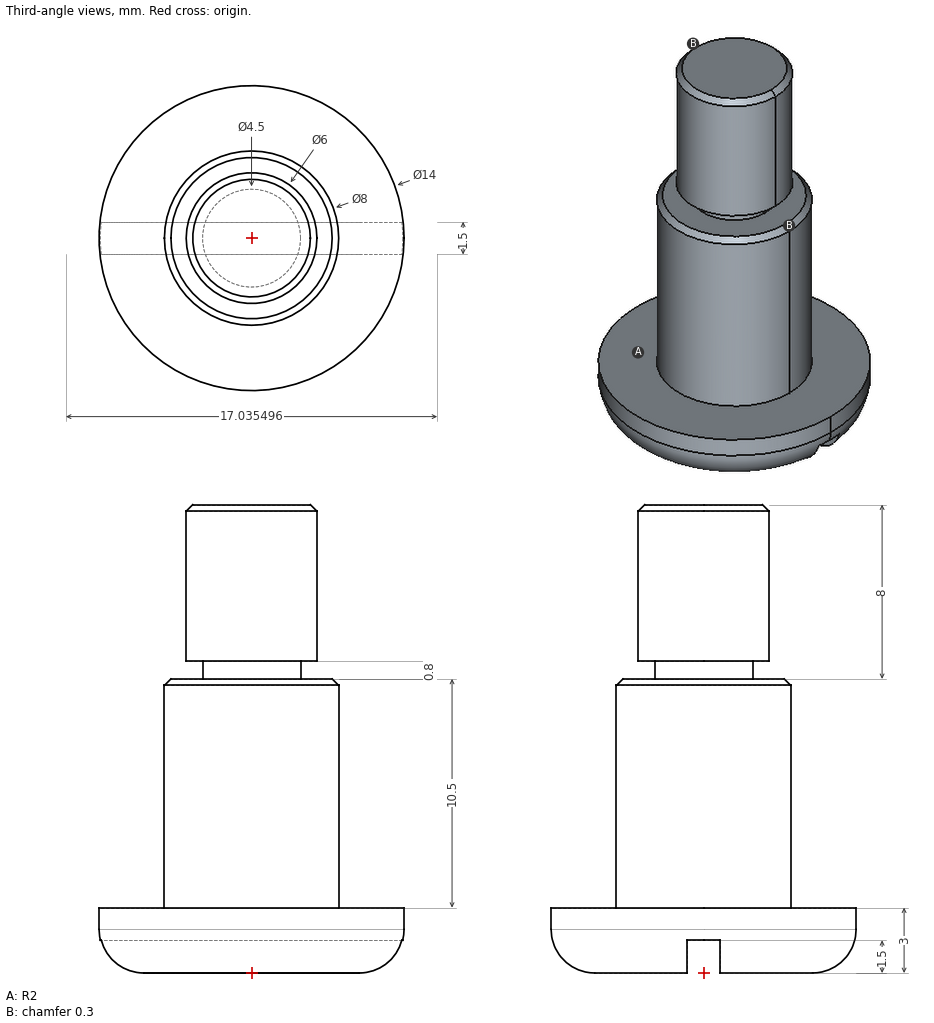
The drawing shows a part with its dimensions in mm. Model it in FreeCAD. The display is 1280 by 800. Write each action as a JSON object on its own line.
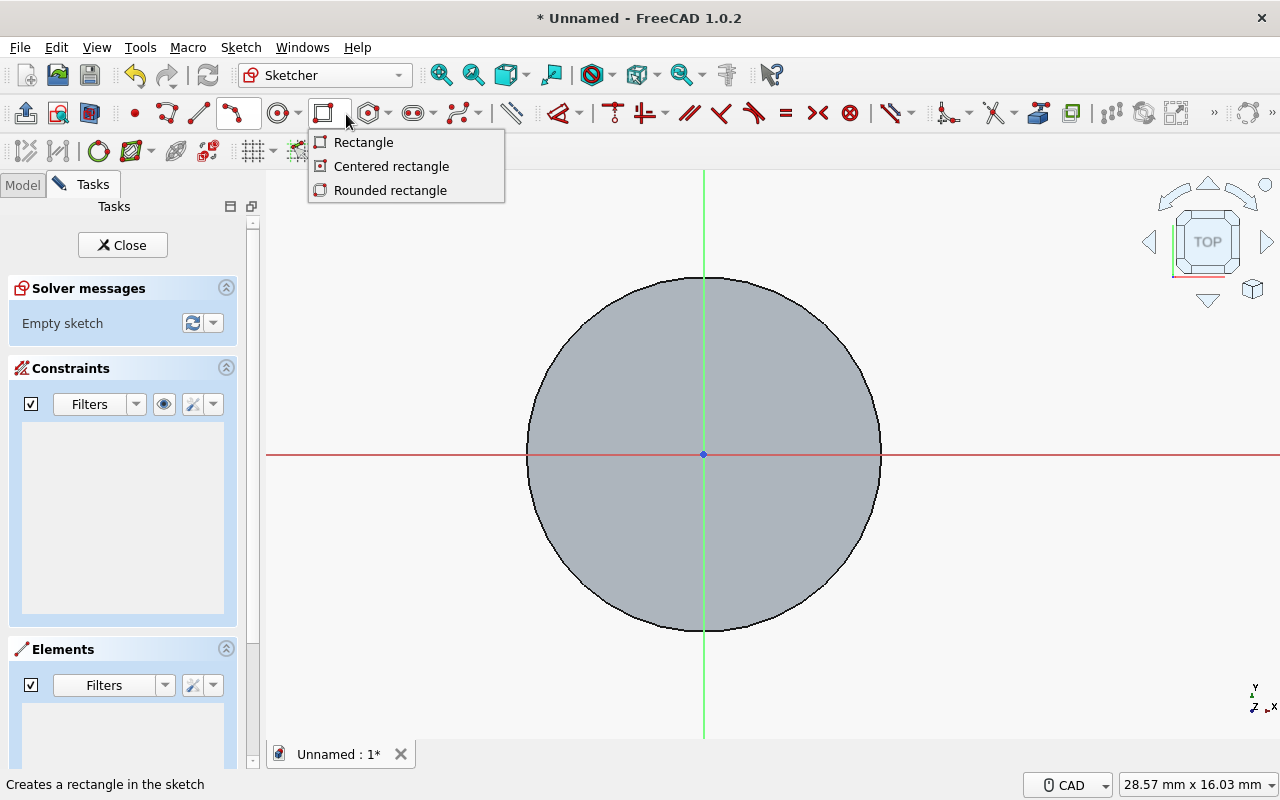
{"action": "left_click", "coordinate": [406, 166]}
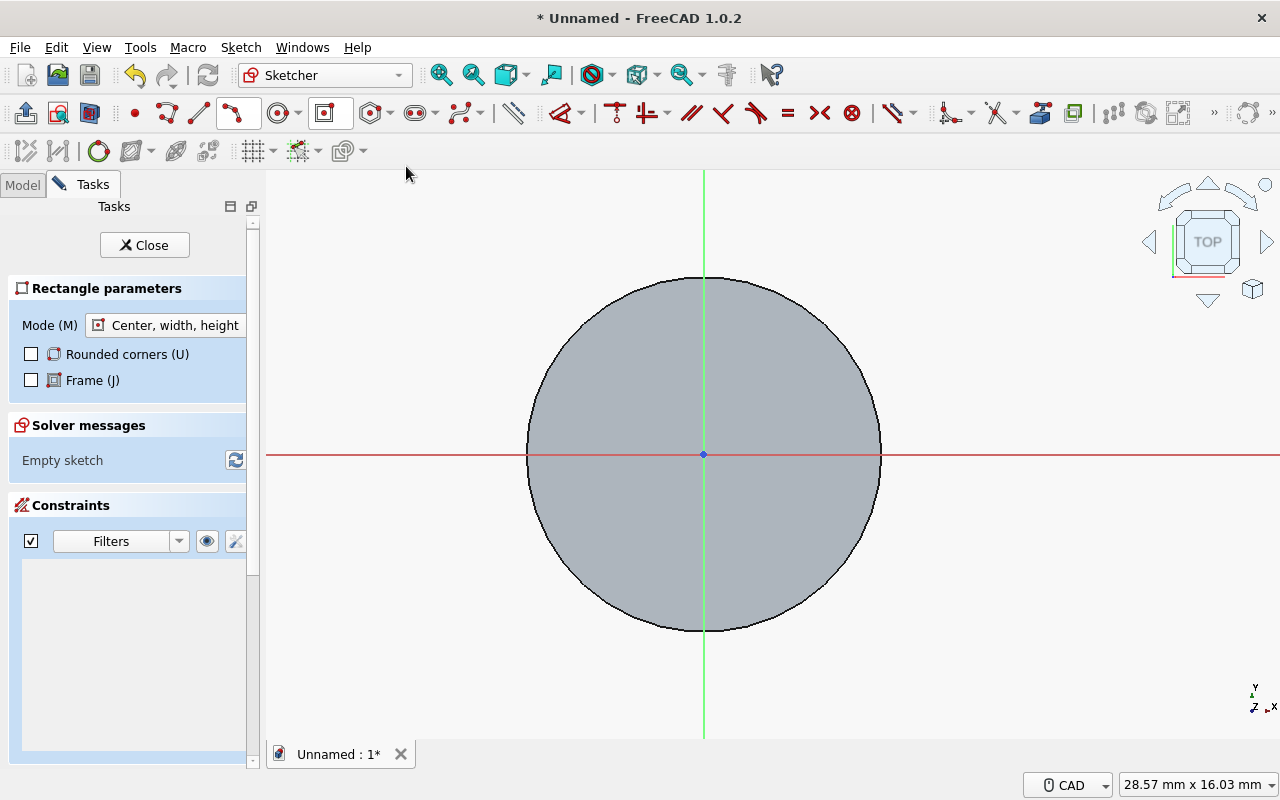
{"action": "left_click", "coordinate": [704, 454]}
{"action": "left_click", "coordinate": [1006, 428]}
{"action": "key", "text": "Escape"}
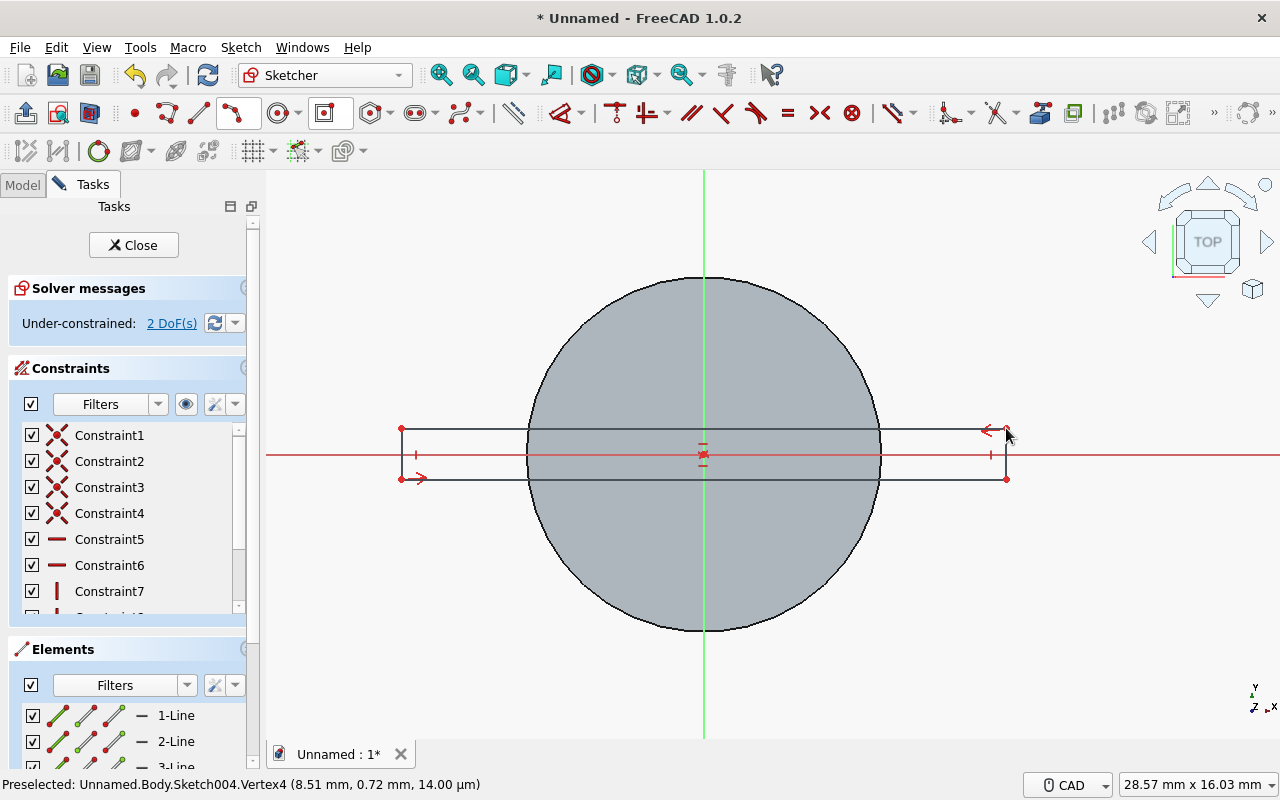
{"action": "left_click", "coordinate": [560, 114]}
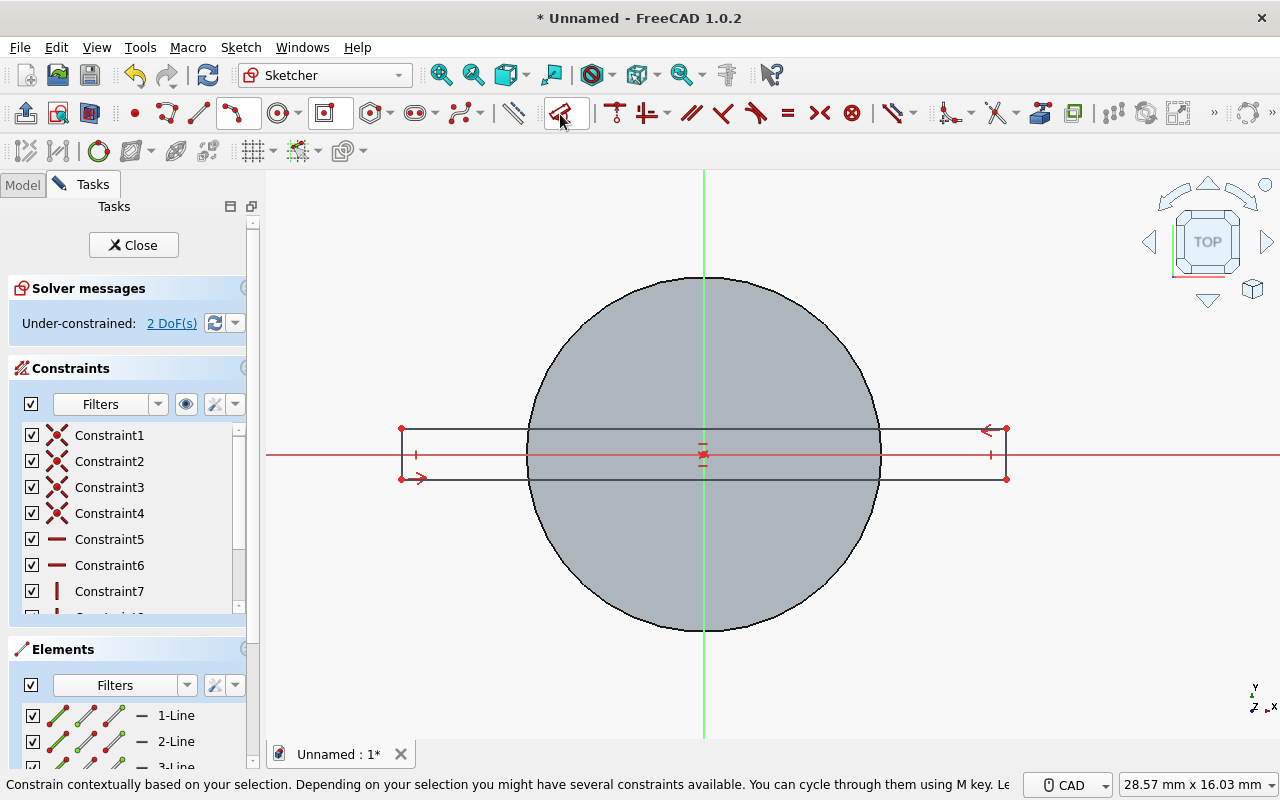
{"action": "scroll", "coordinate": [1006, 465], "scroll_direction": "up", "scroll_amount": 2}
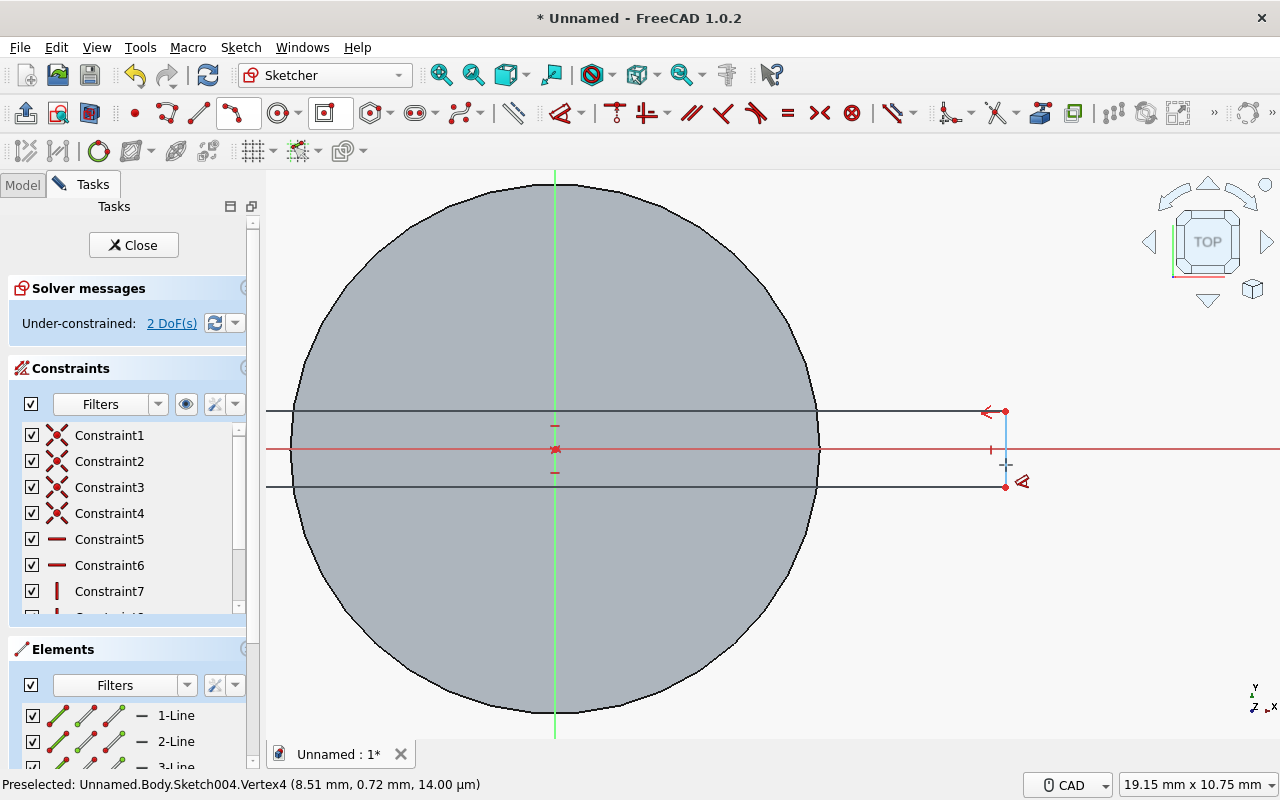
{"action": "left_click", "coordinate": [1006, 464]}
{"action": "left_click", "coordinate": [1040, 432]}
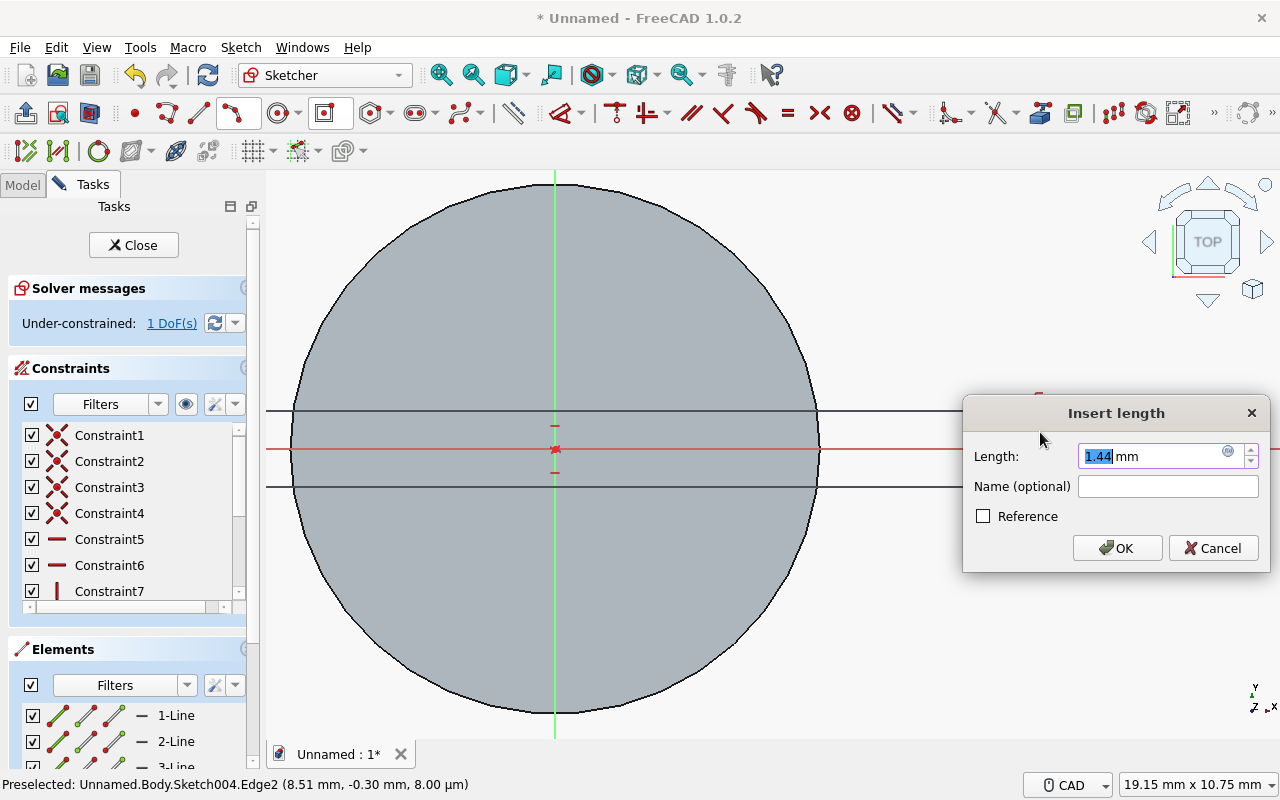
{"action": "type", "text": "1.5"}
{"action": "key", "text": "Return"}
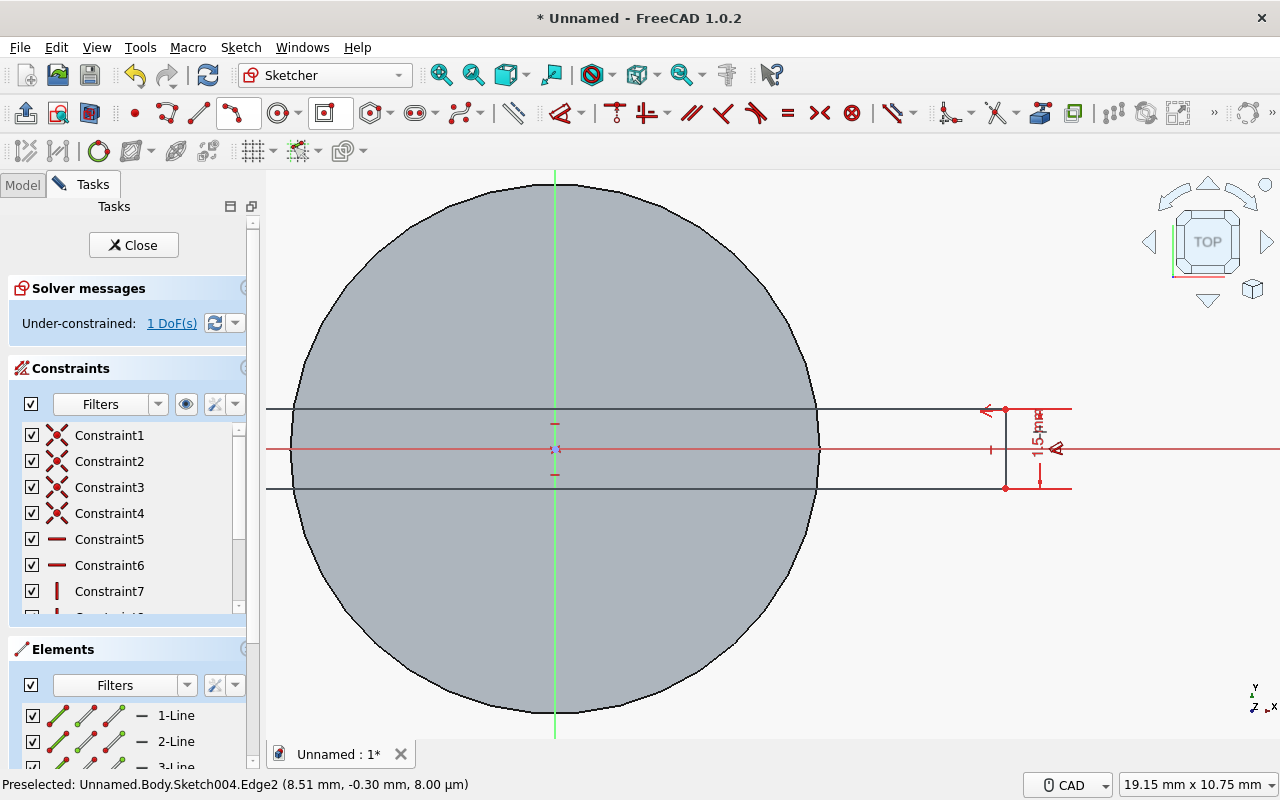
{"action": "left_click", "coordinate": [375, 489]}
{"action": "left_click", "coordinate": [650, 523]}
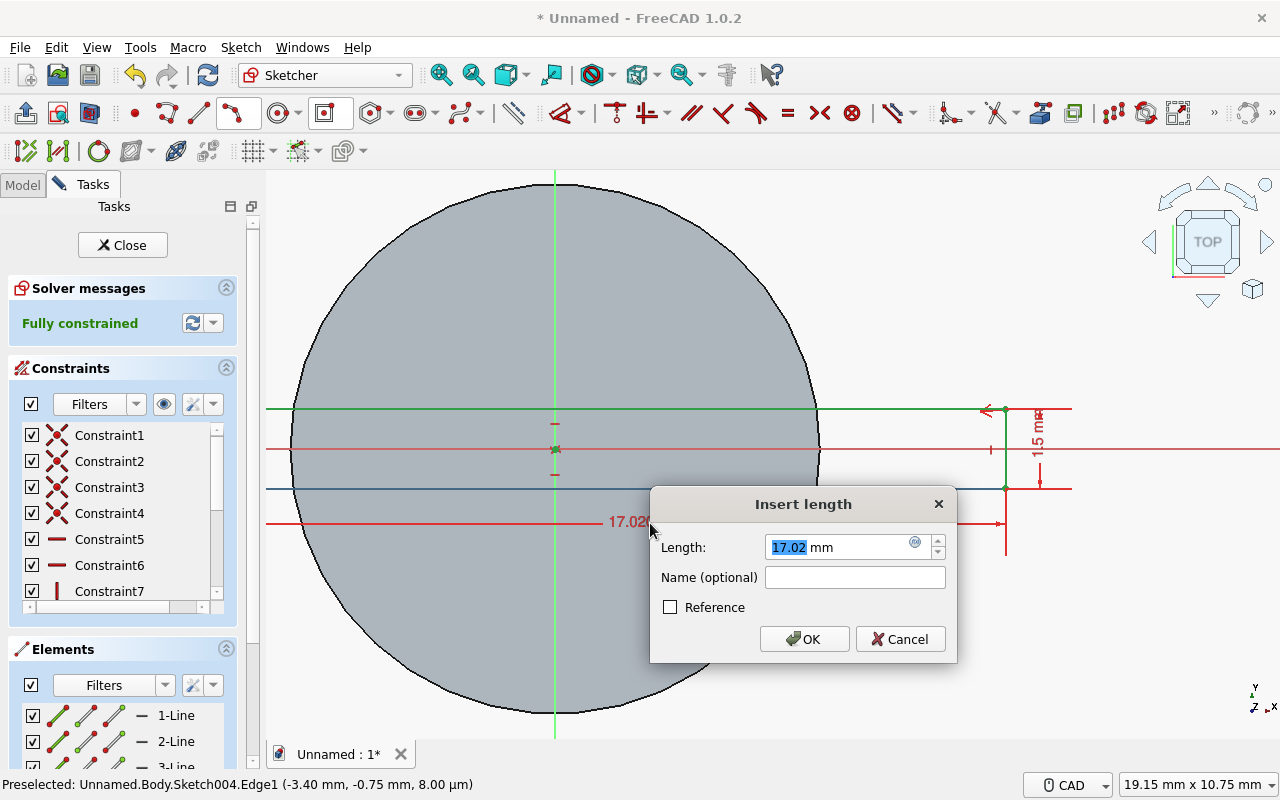
{"action": "type", "text": "17.035496"}
{"action": "key", "text": "Return"}
{"action": "key", "text": "Escape"}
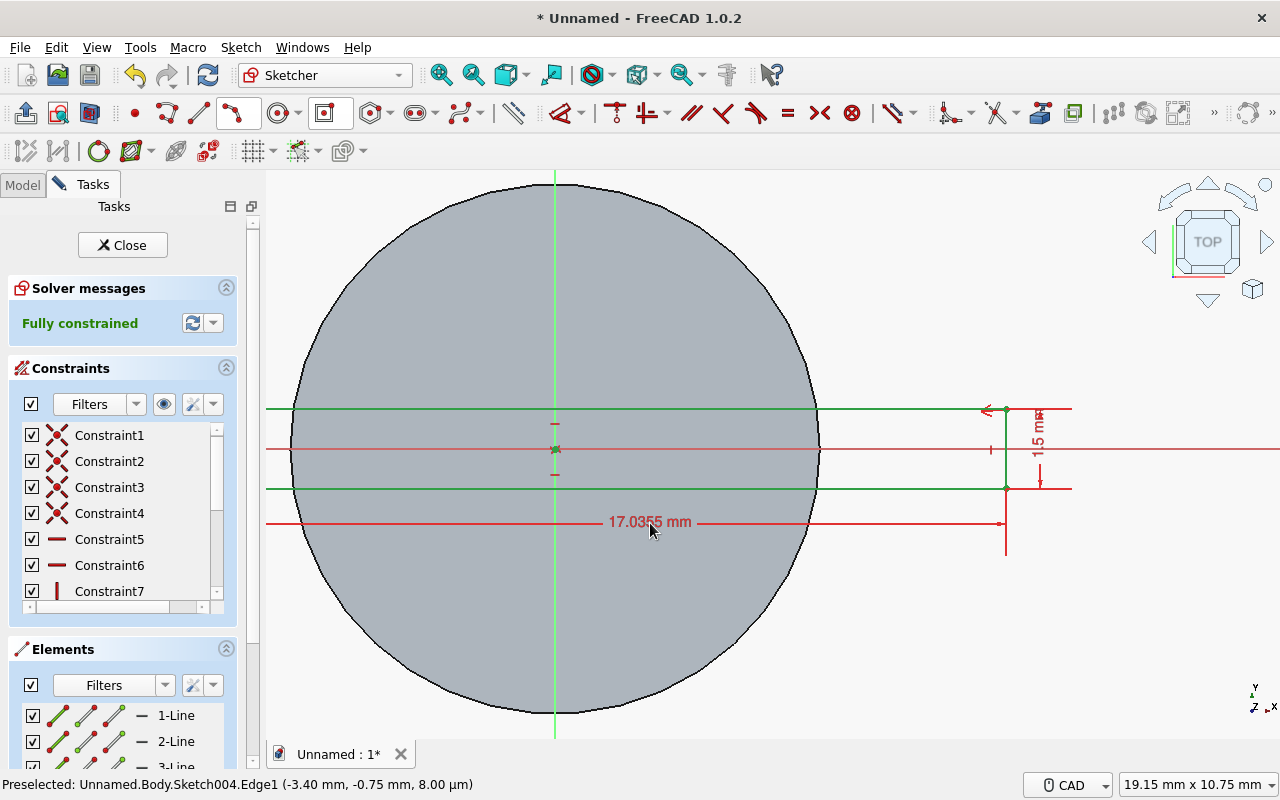
{"action": "left_click", "coordinate": [123, 245]}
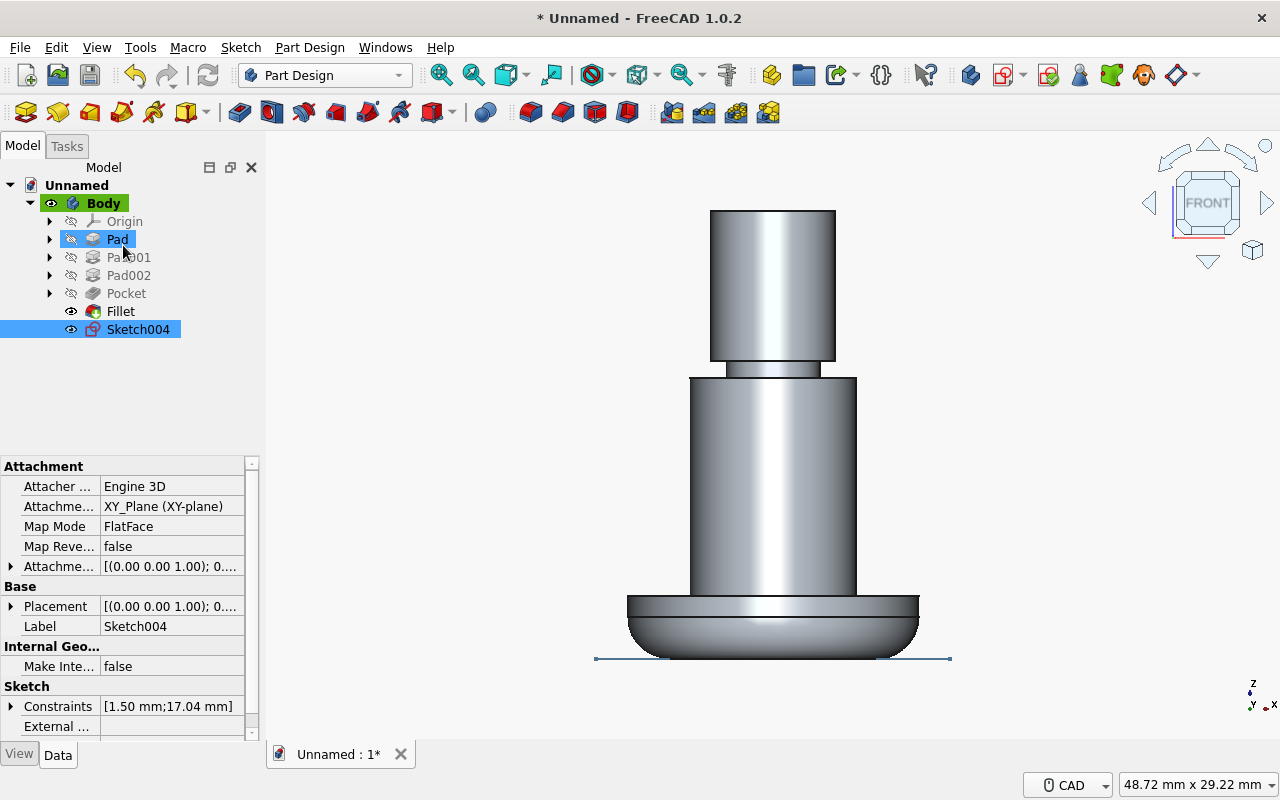
{"action": "left_click", "coordinate": [240, 112]}